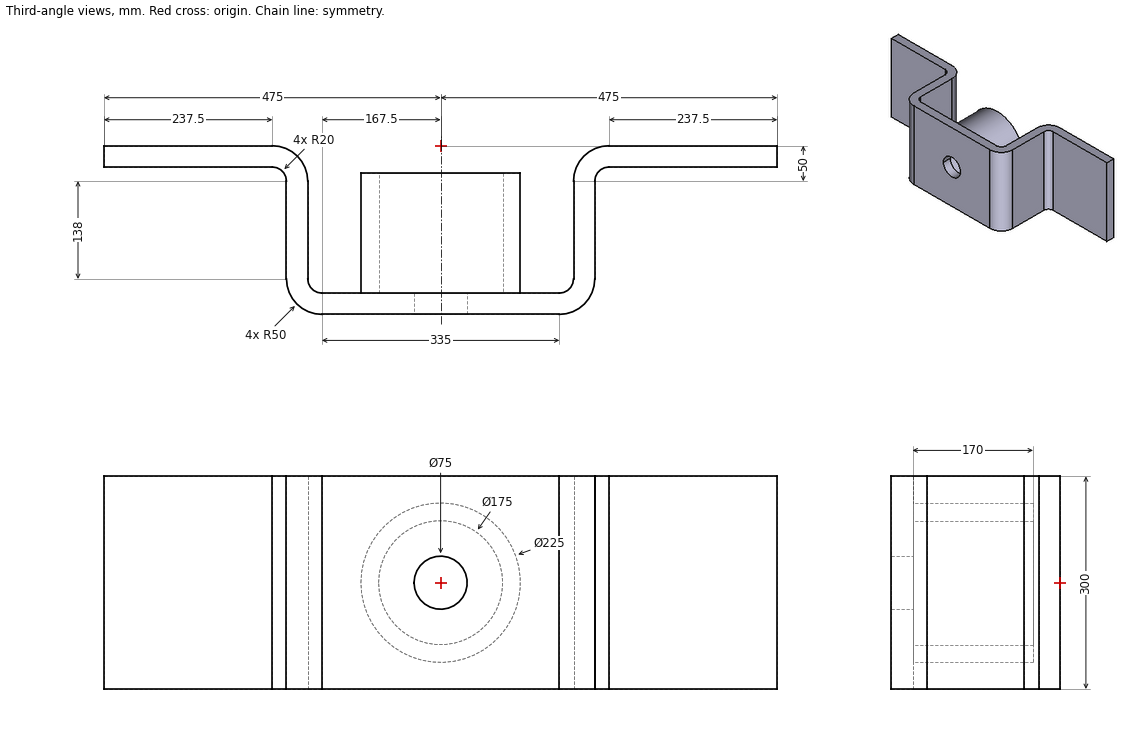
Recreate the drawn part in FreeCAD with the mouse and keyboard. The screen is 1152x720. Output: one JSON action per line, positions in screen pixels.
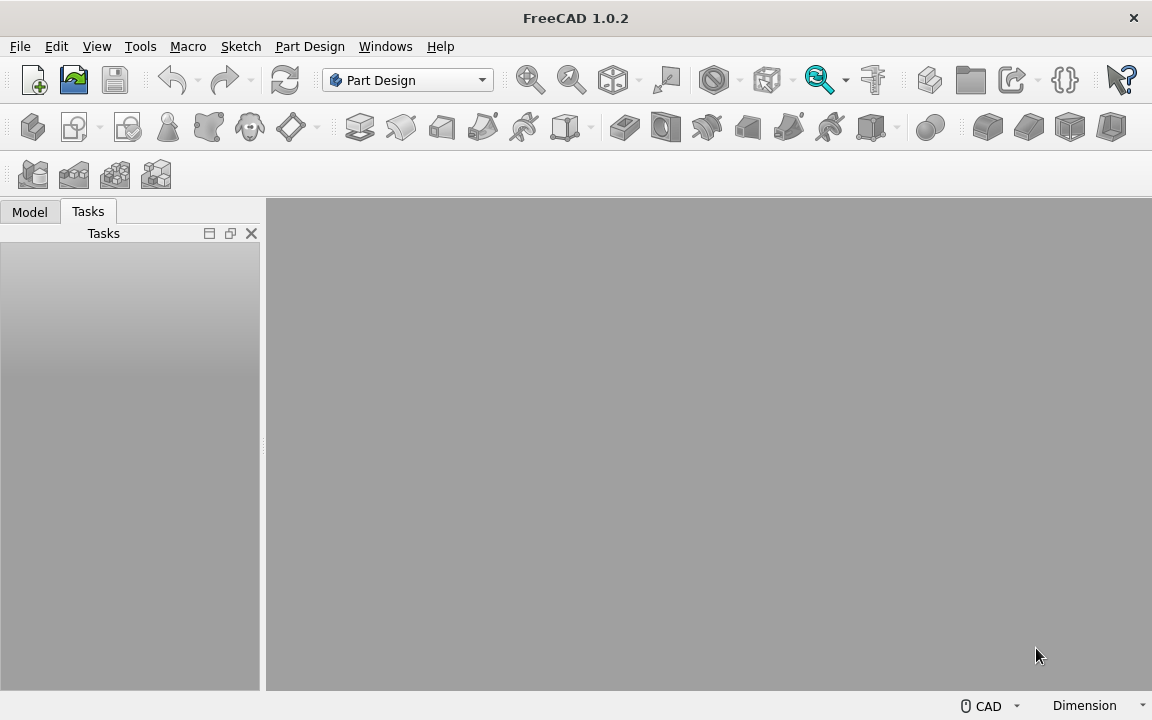
{"action": "key", "text": "ctrl+n"}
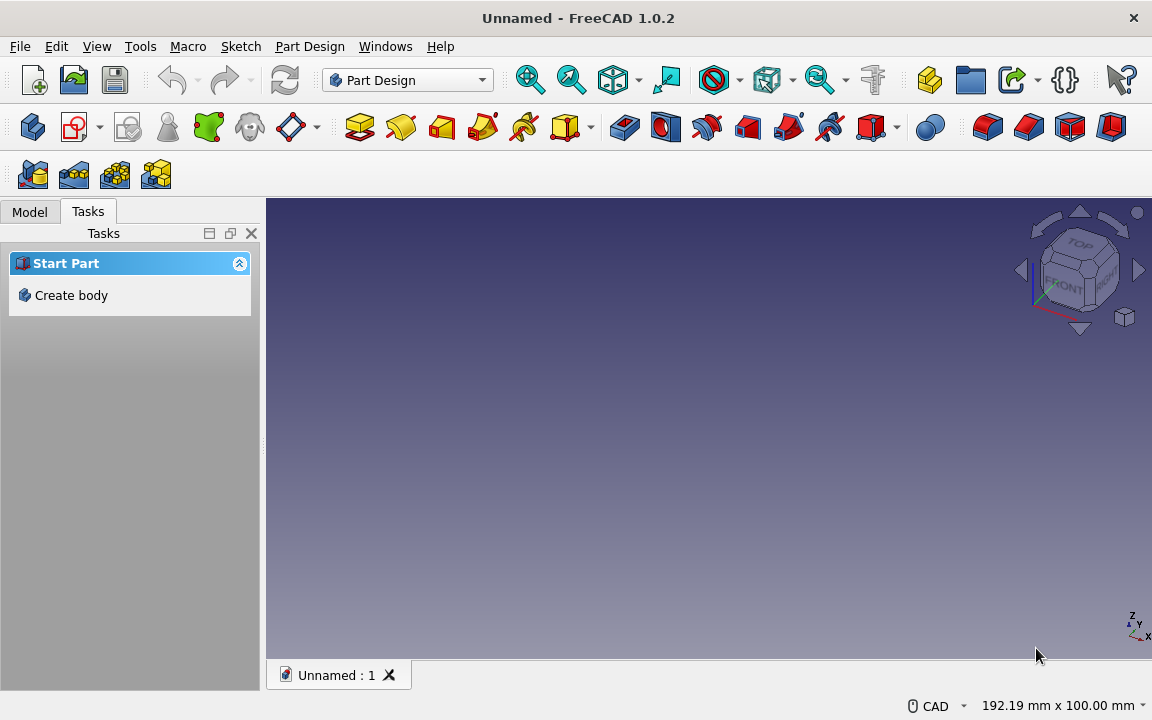
{"action": "left_click", "coordinate": [74, 128]}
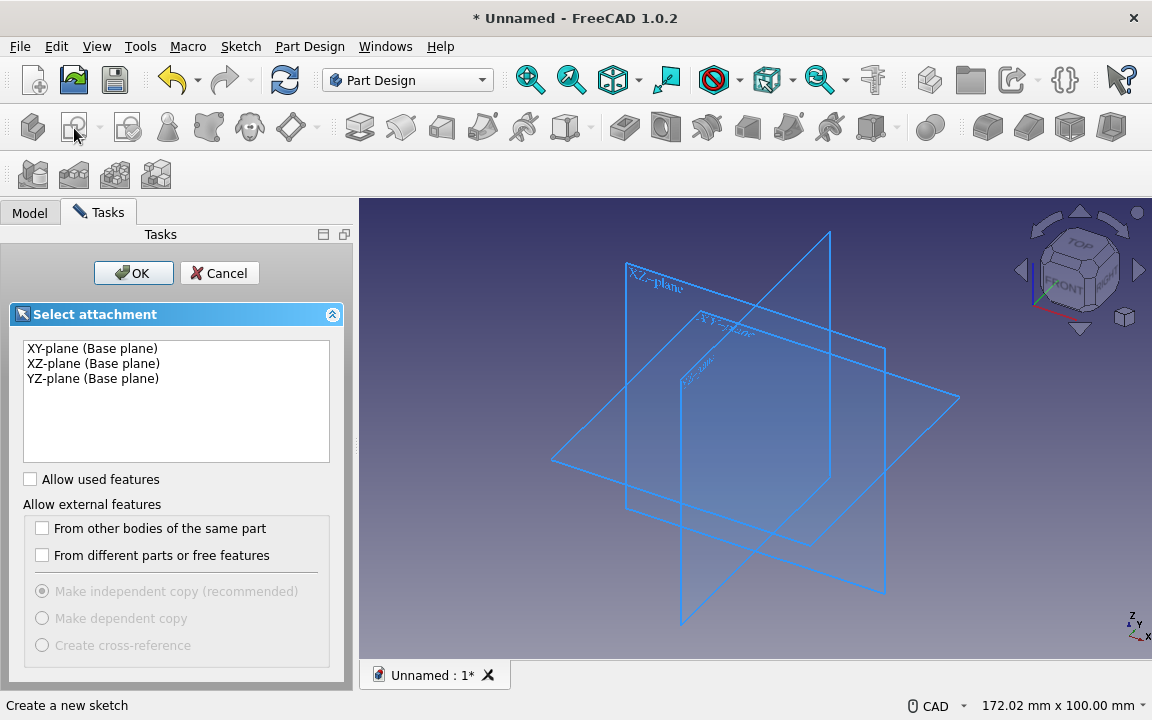
{"action": "left_click", "coordinate": [84, 348]}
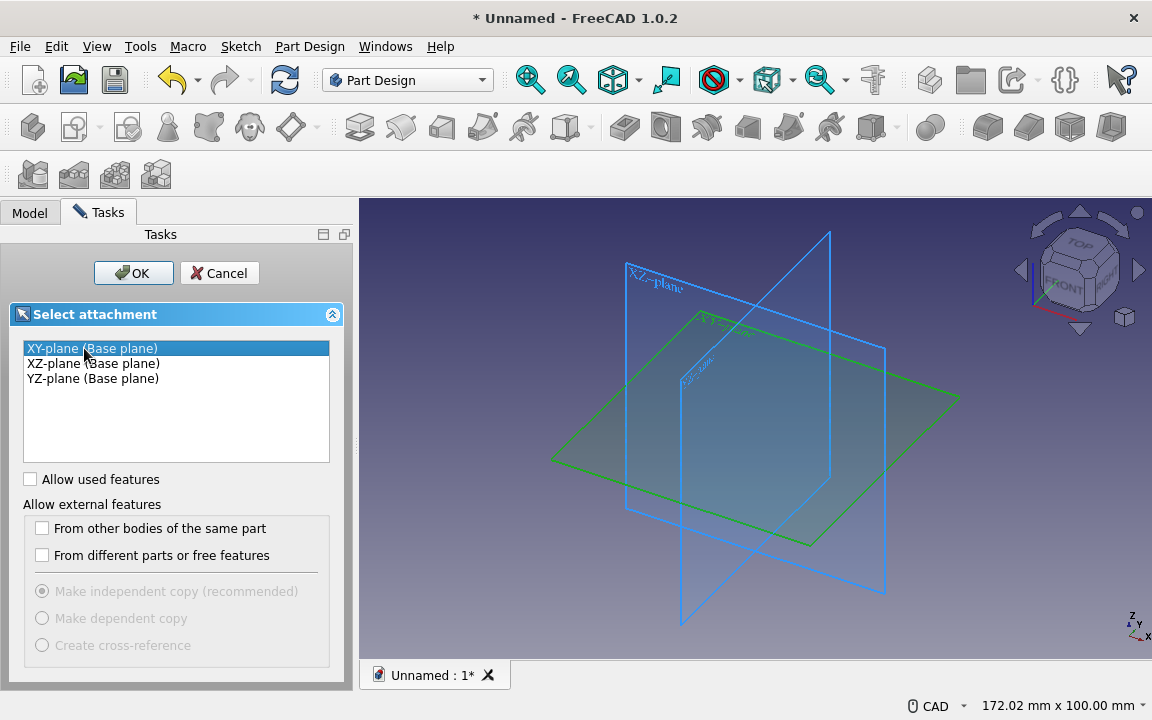
{"action": "left_click", "coordinate": [134, 273]}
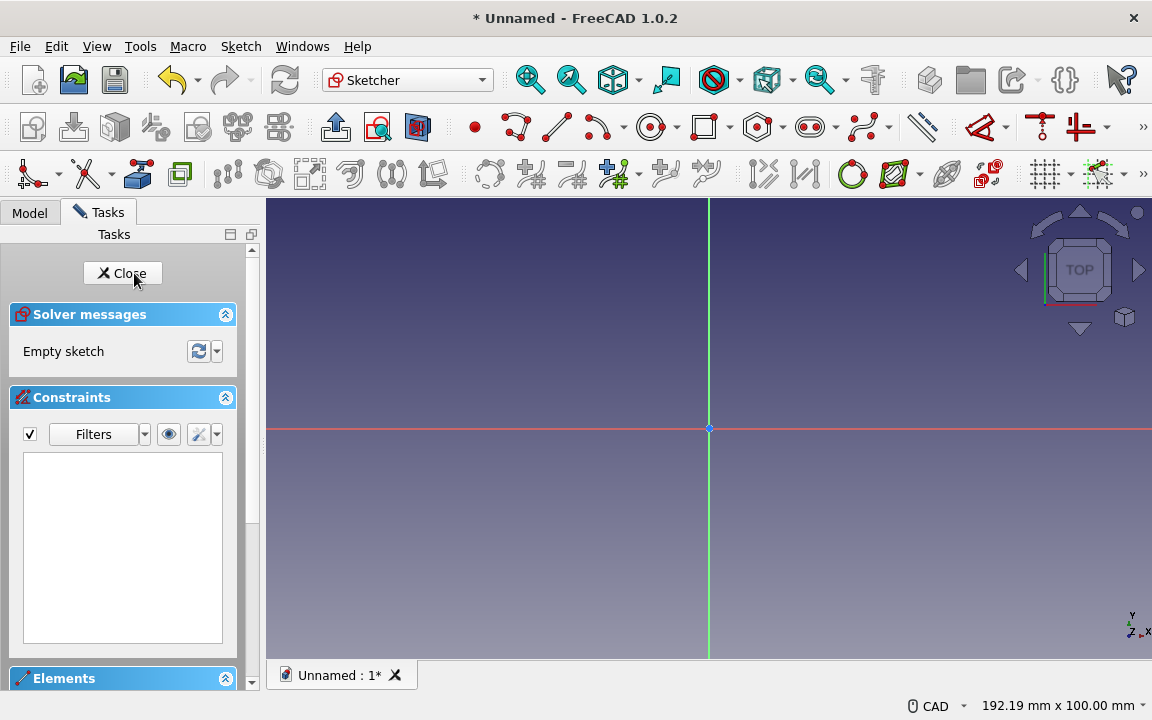
{"action": "scroll", "coordinate": [632, 360], "scroll_direction": "down", "scroll_amount": 11}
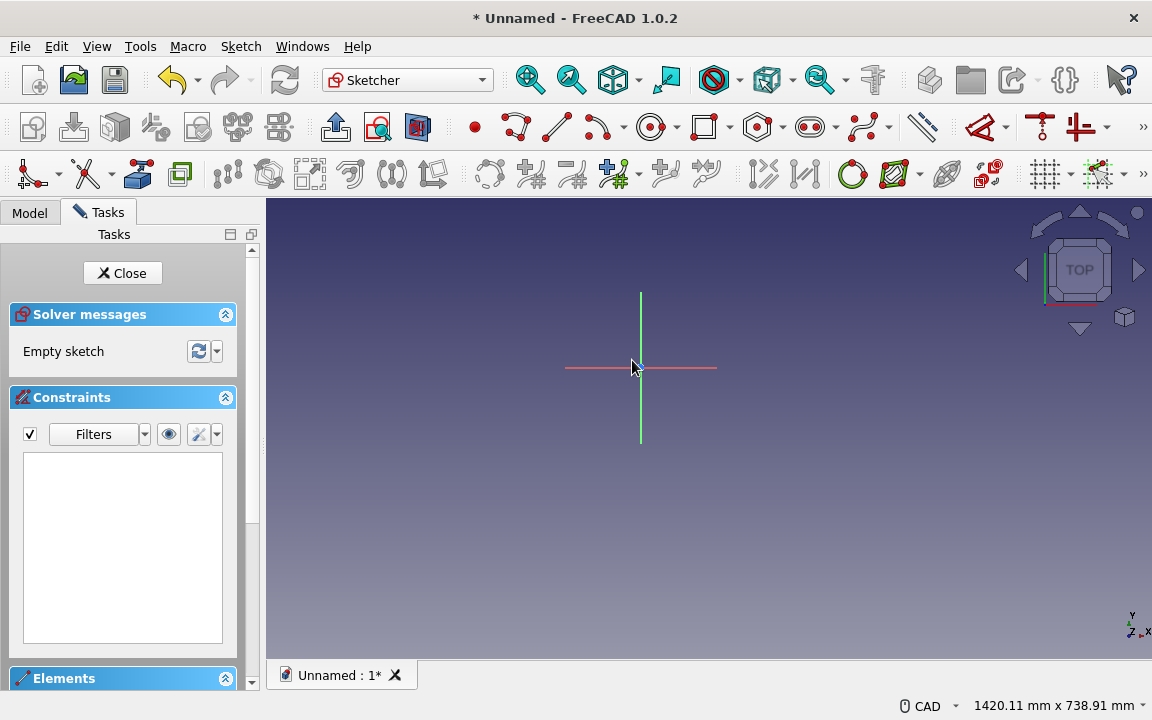
{"action": "key", "text": "g m"}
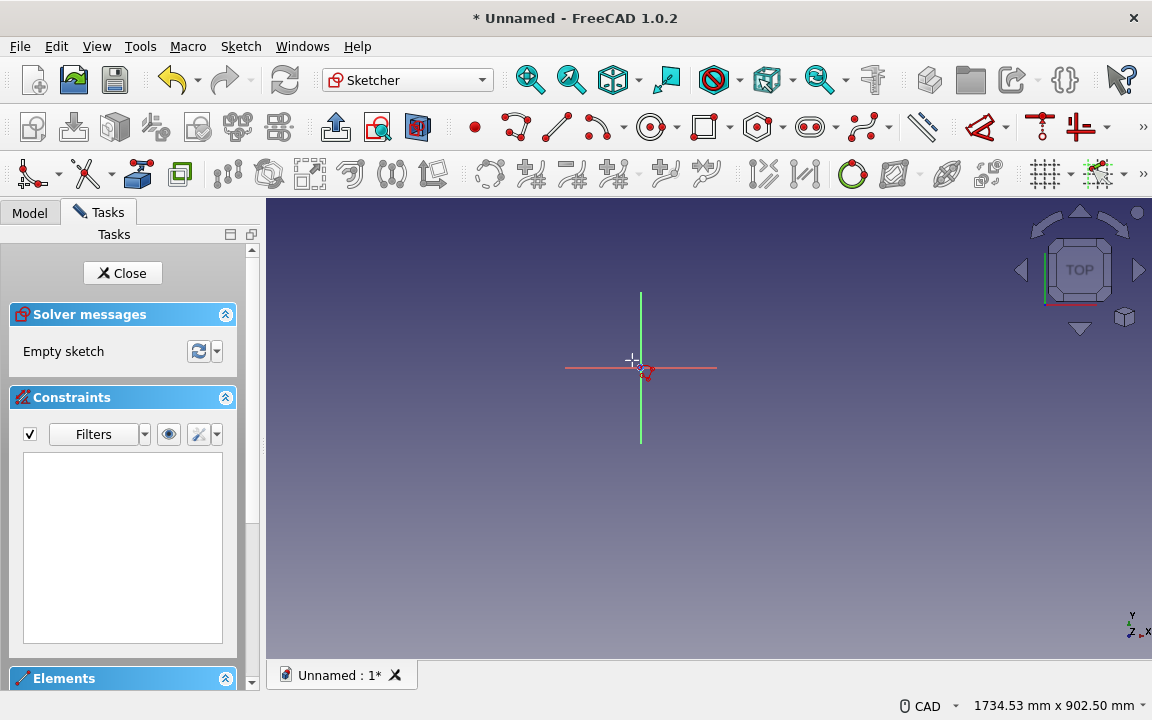
{"action": "left_click", "coordinate": [520, 368]}
{"action": "left_click", "coordinate": [398, 377]}
{"action": "left_click", "coordinate": [398, 383]}
{"action": "left_click", "coordinate": [520, 383]}
{"action": "right_click", "coordinate": [520, 383]}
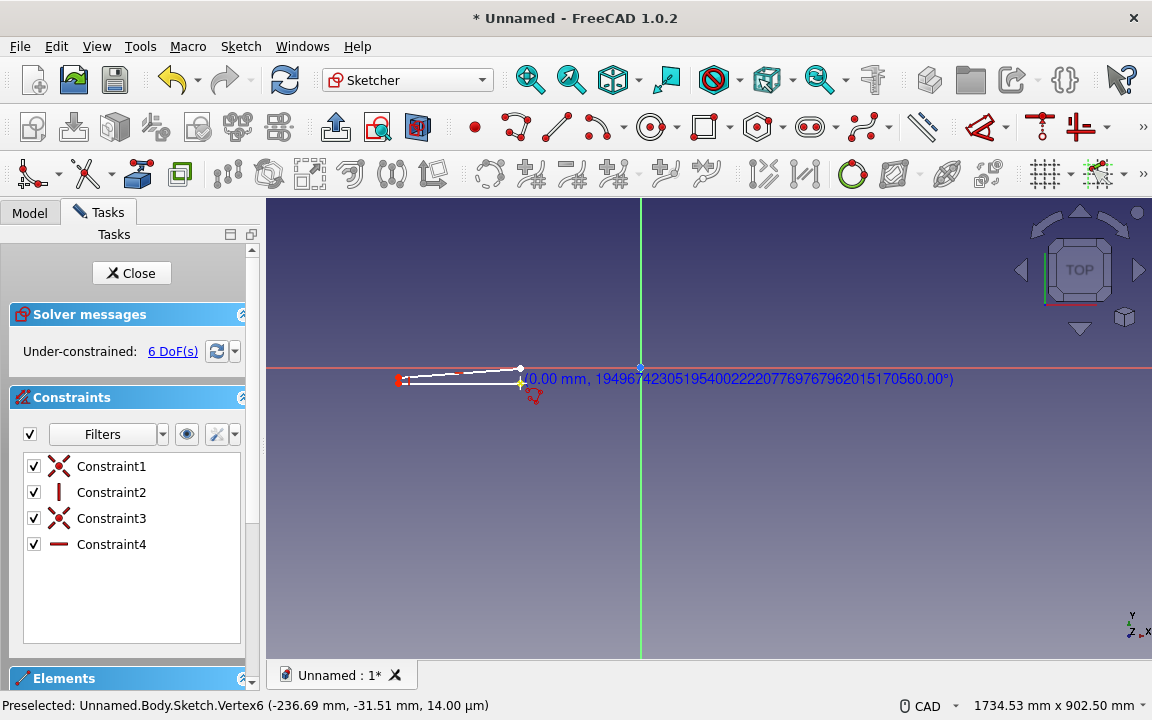
{"action": "left_click", "coordinate": [557, 128]}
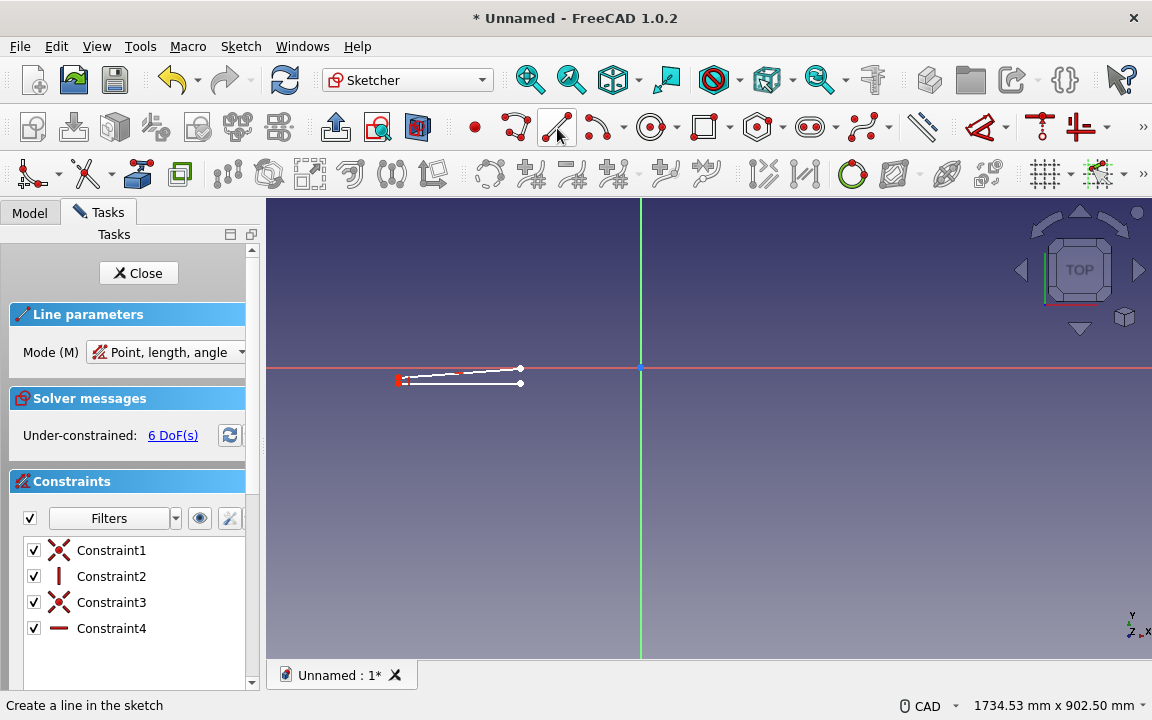
{"action": "left_click", "coordinate": [530, 393]}
{"action": "left_click", "coordinate": [530, 464]}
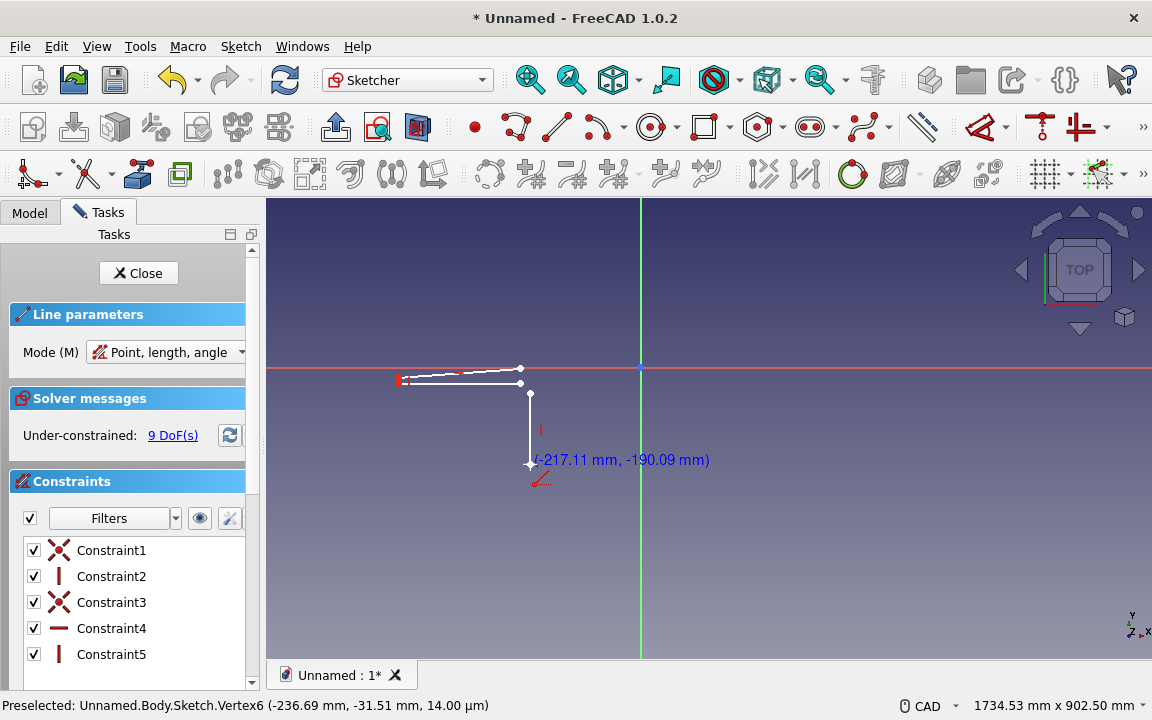
{"action": "left_click", "coordinate": [555, 489]}
{"action": "left_click", "coordinate": [726, 489]}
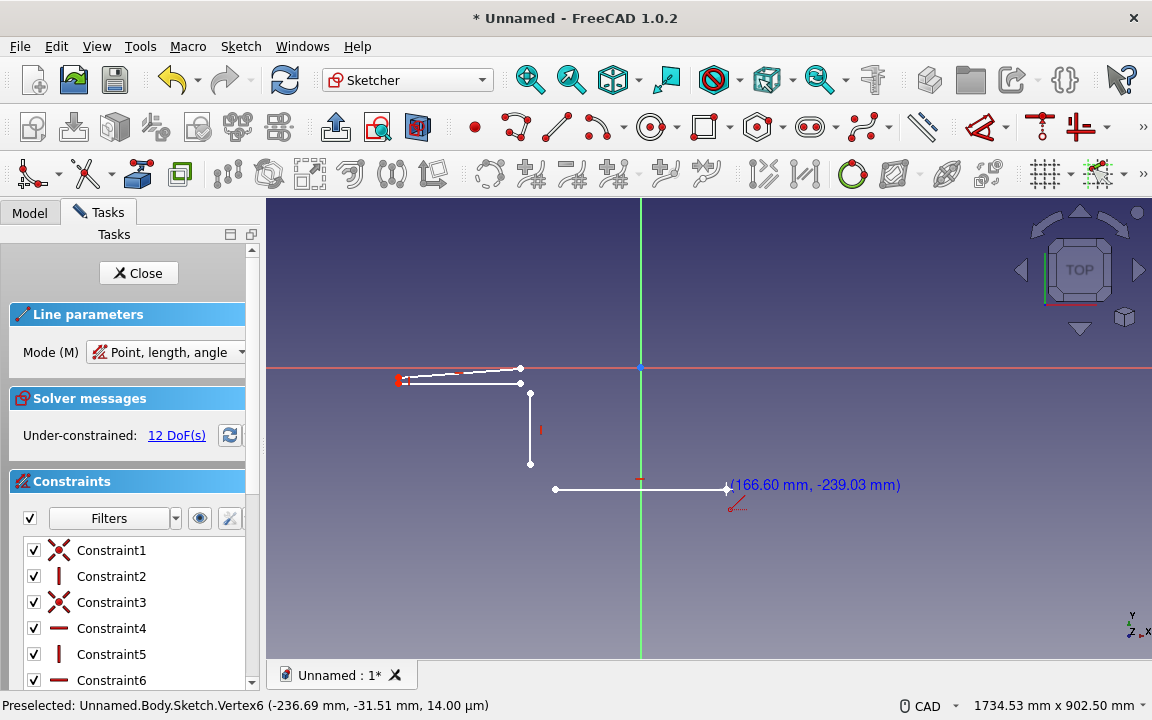
{"action": "left_click", "coordinate": [752, 464]}
{"action": "left_click", "coordinate": [752, 393]}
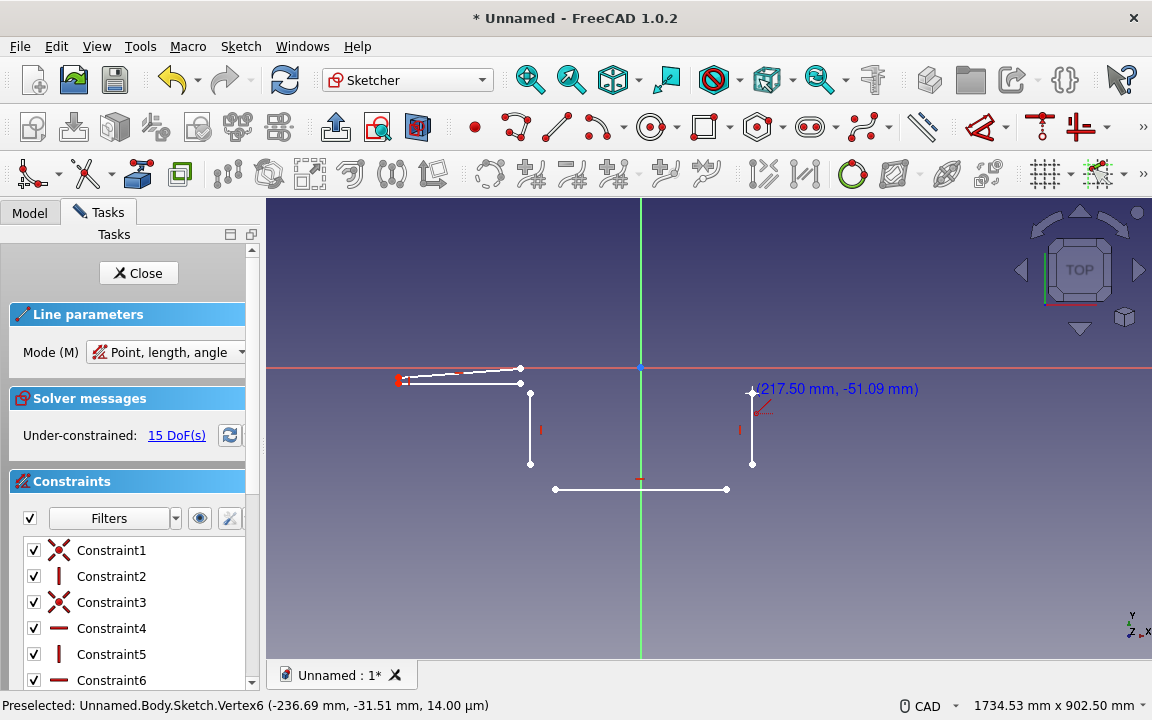
{"action": "key", "text": "g m"}